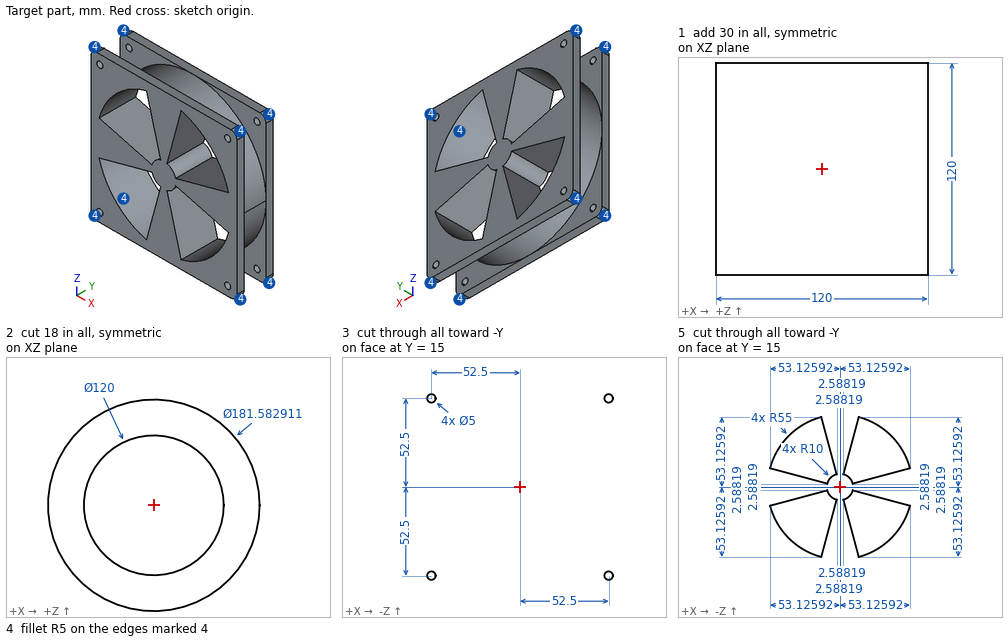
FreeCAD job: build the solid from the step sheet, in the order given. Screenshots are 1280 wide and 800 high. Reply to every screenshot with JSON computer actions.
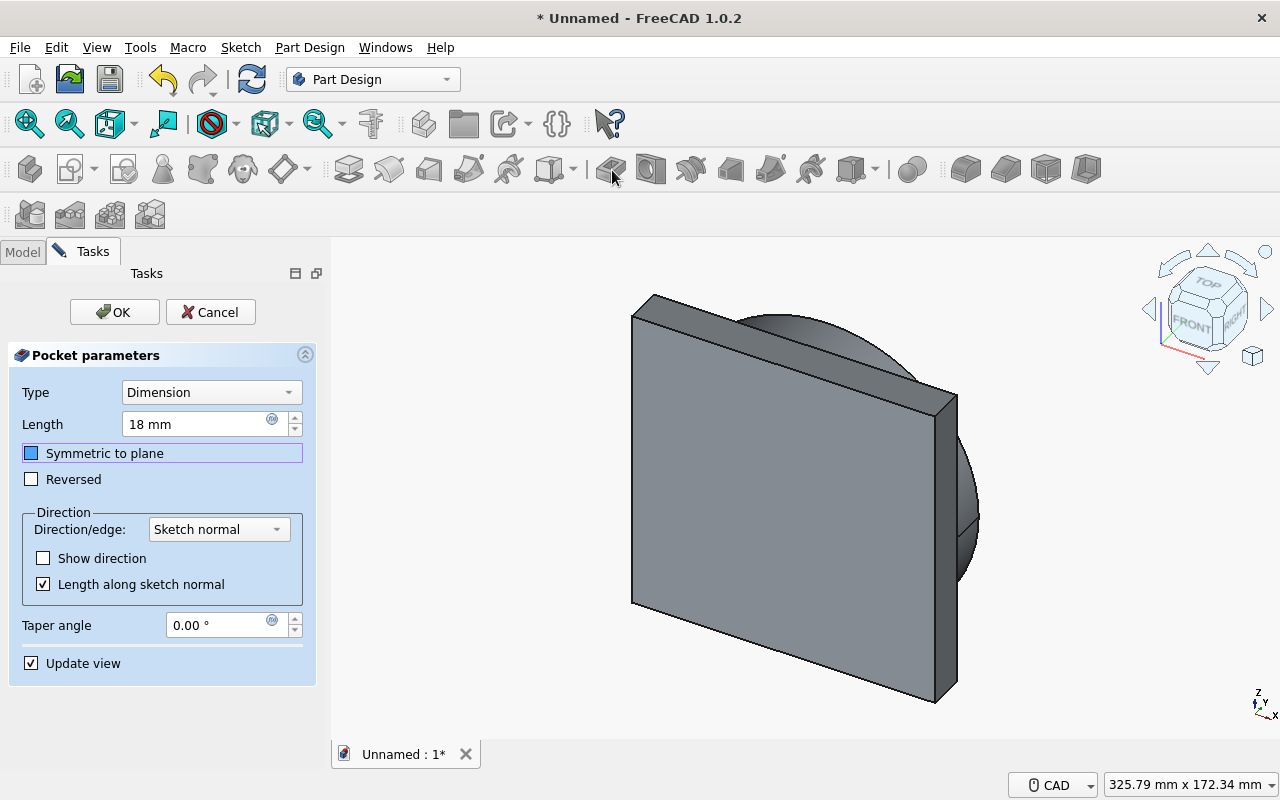
{"action": "left_click", "coordinate": [30, 453]}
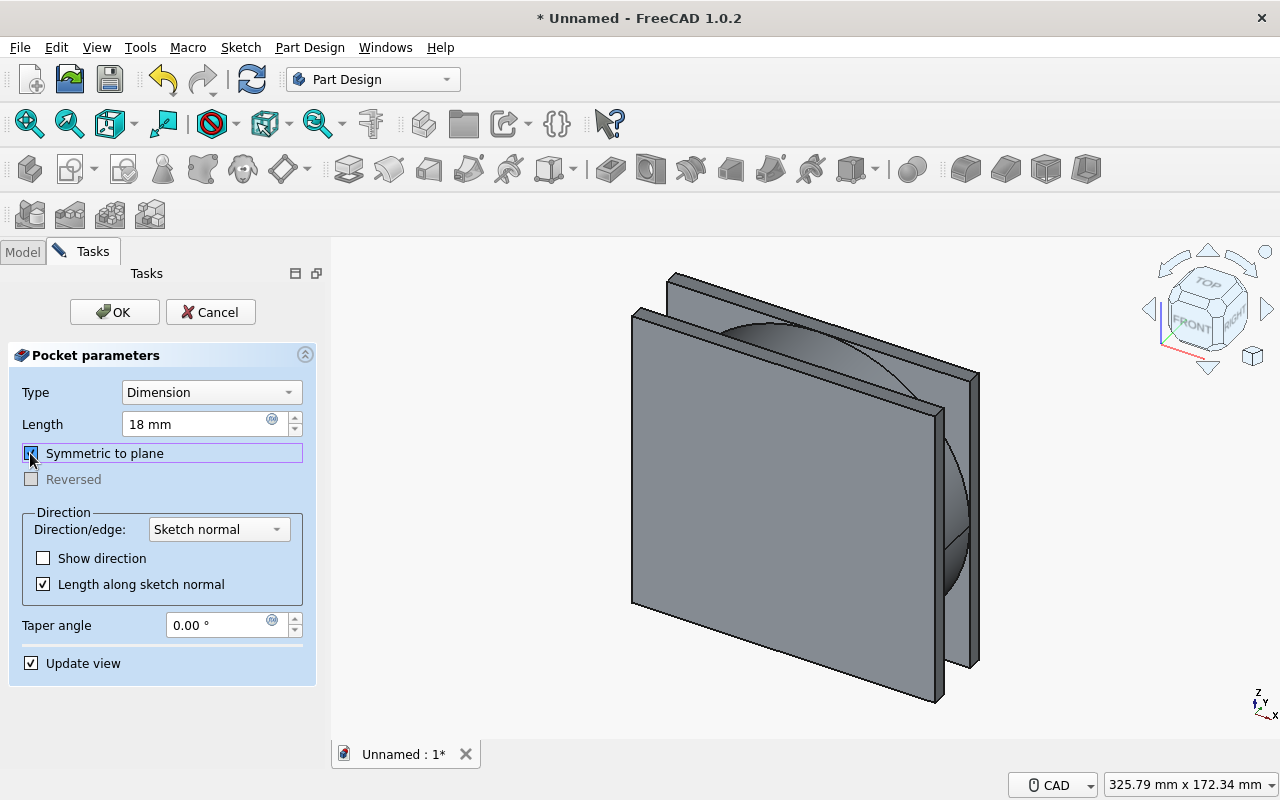
{"action": "left_click", "coordinate": [115, 312]}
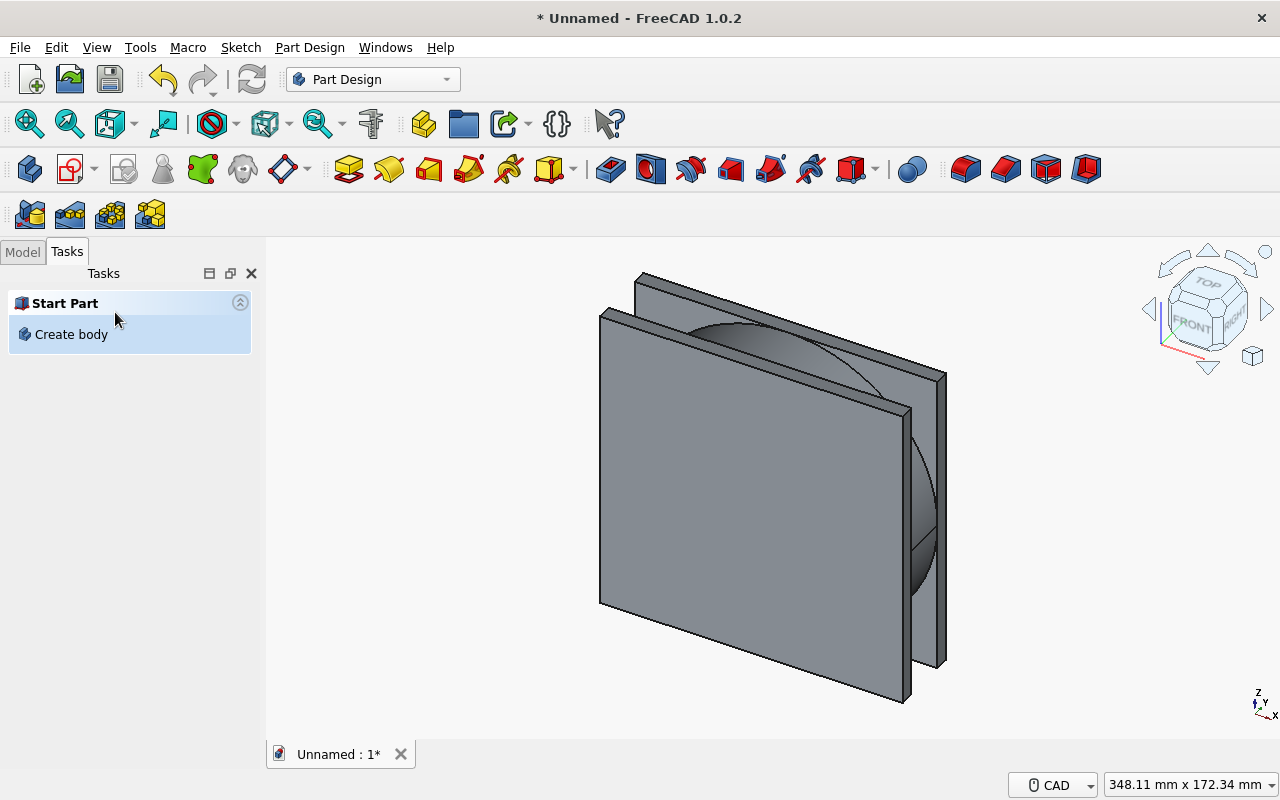
{"action": "key", "text": "4"}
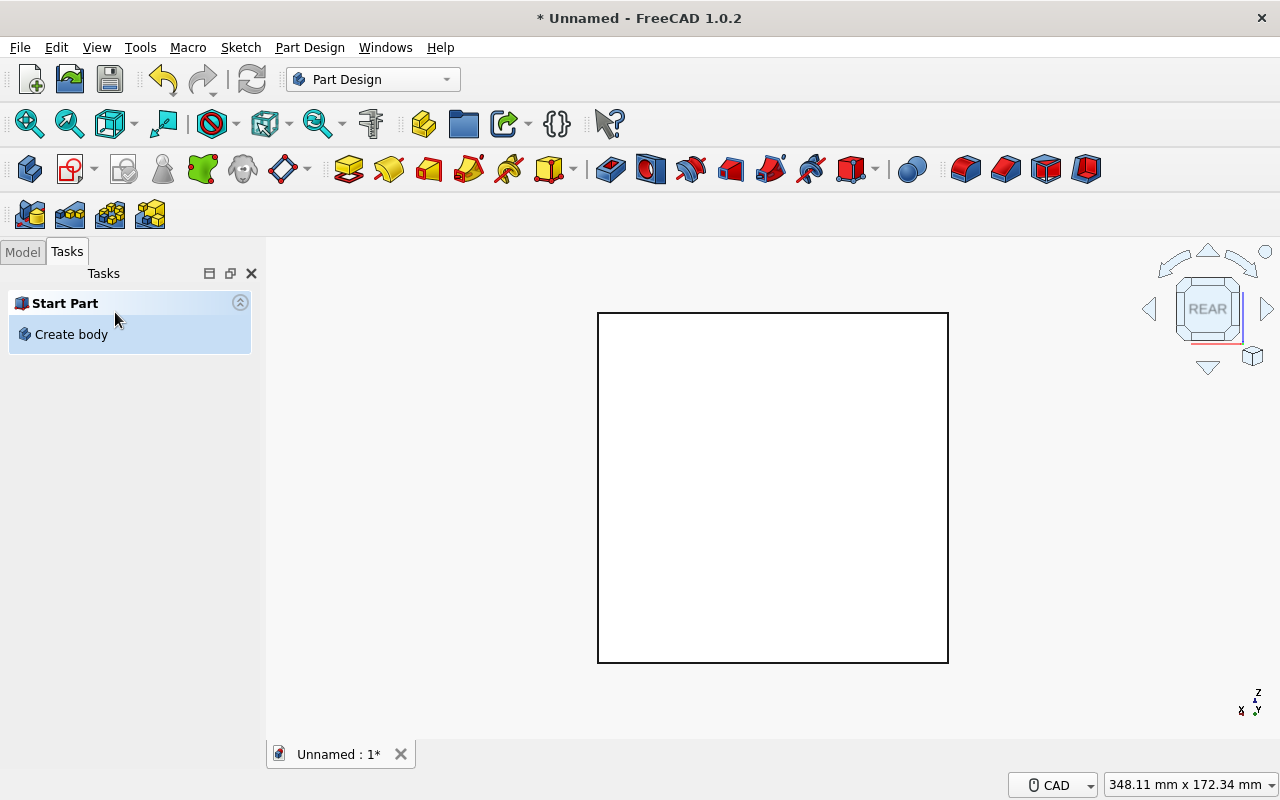
{"action": "left_click", "coordinate": [773, 487]}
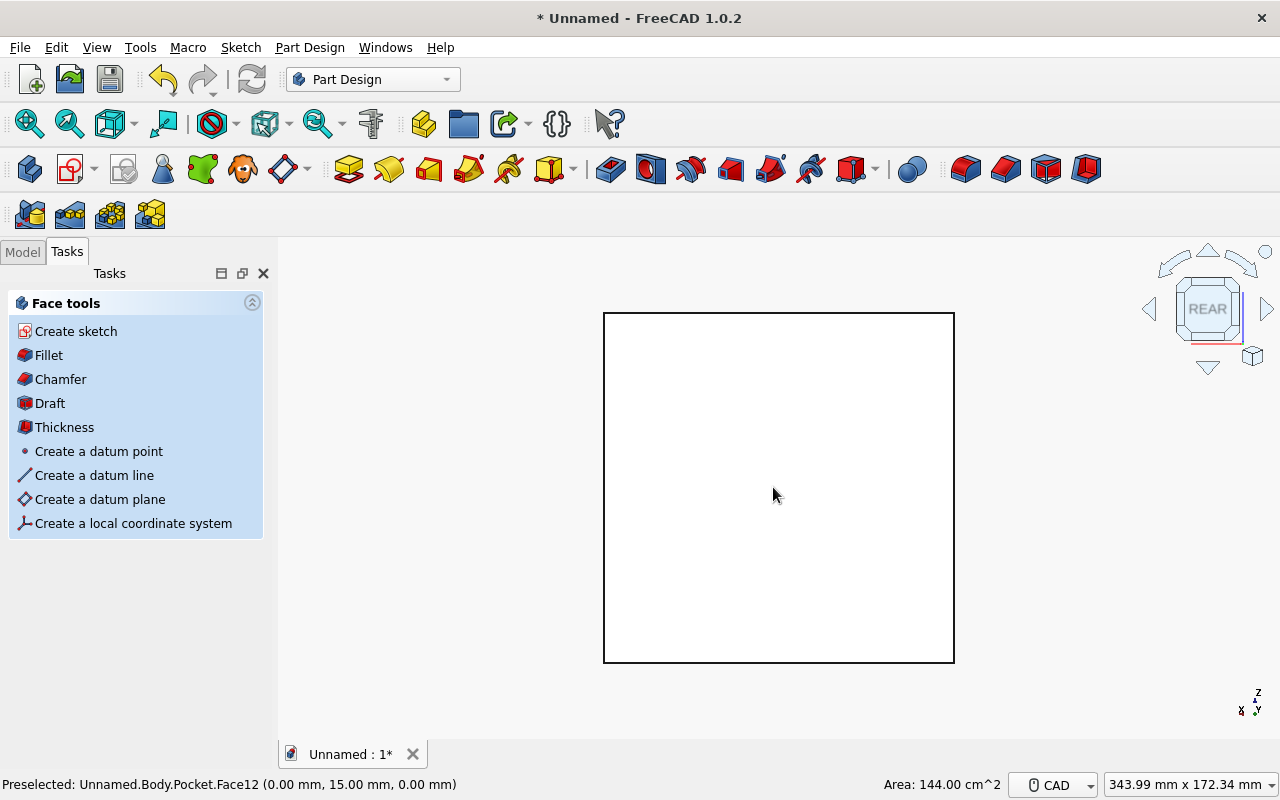
{"action": "left_click", "coordinate": [70, 170]}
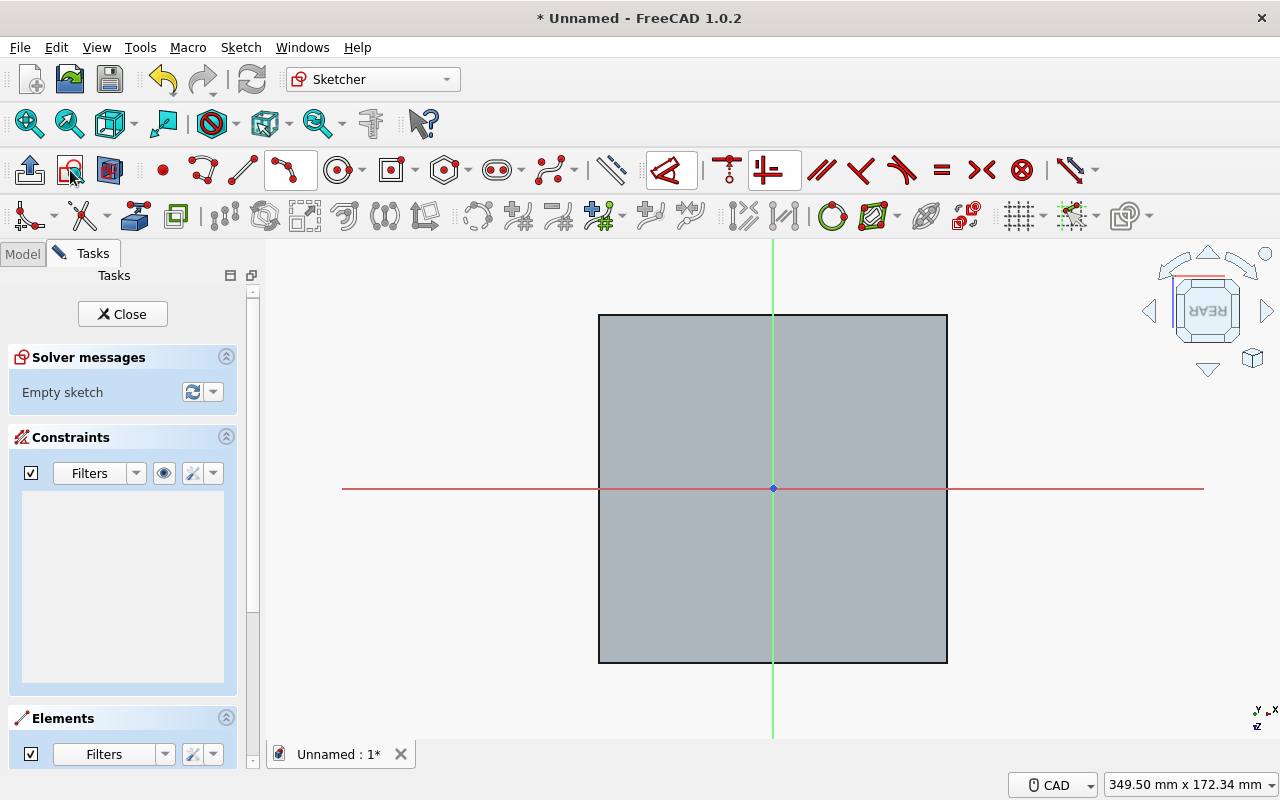
{"action": "left_click", "coordinate": [338, 170]}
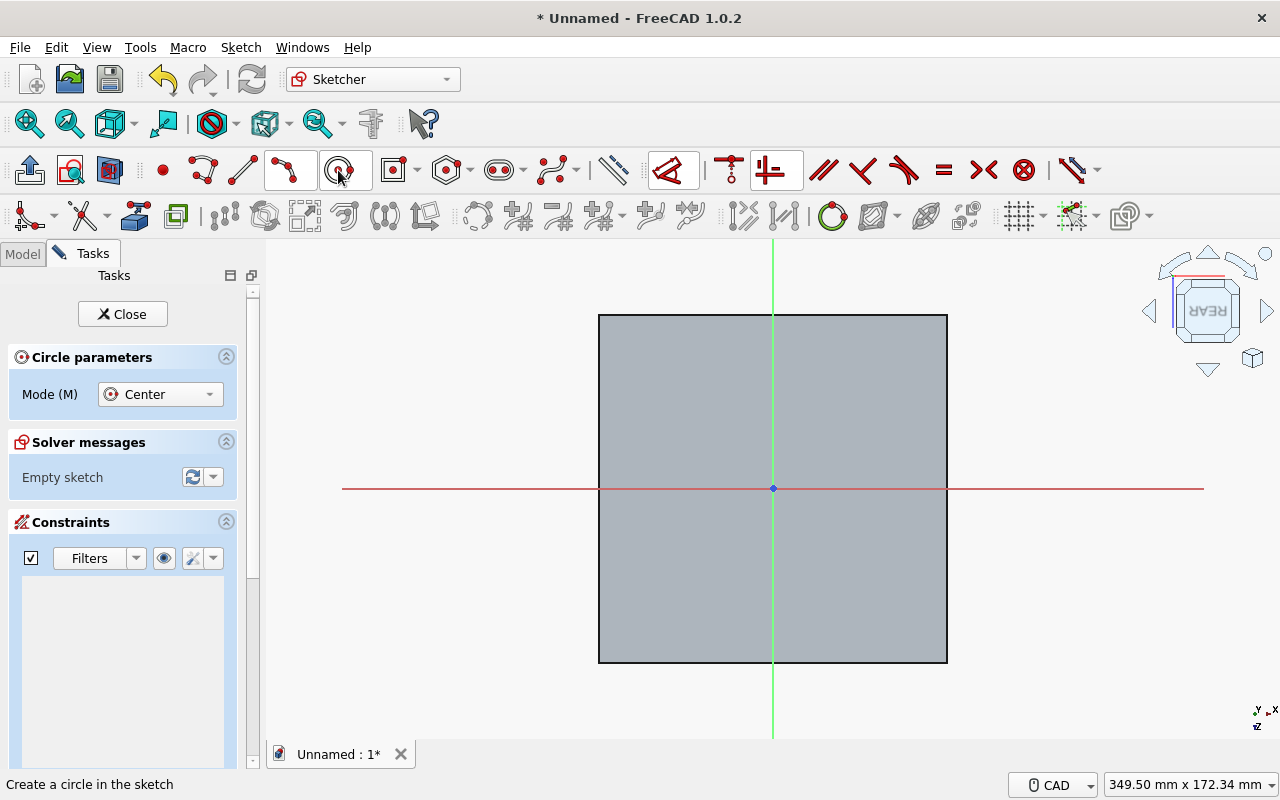
{"action": "scroll", "coordinate": [621, 337], "scroll_direction": "up", "scroll_amount": 6}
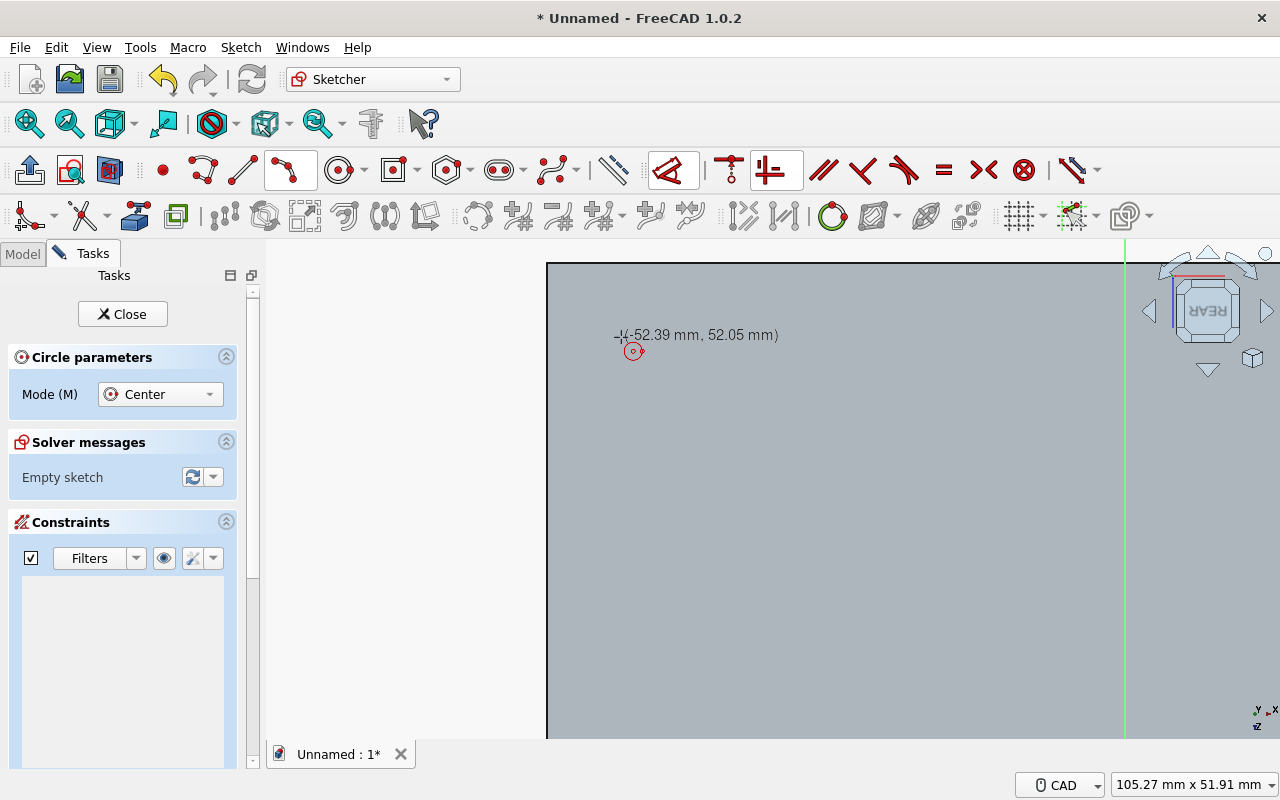
{"action": "left_click", "coordinate": [619, 335]}
{"action": "left_click", "coordinate": [636, 318]}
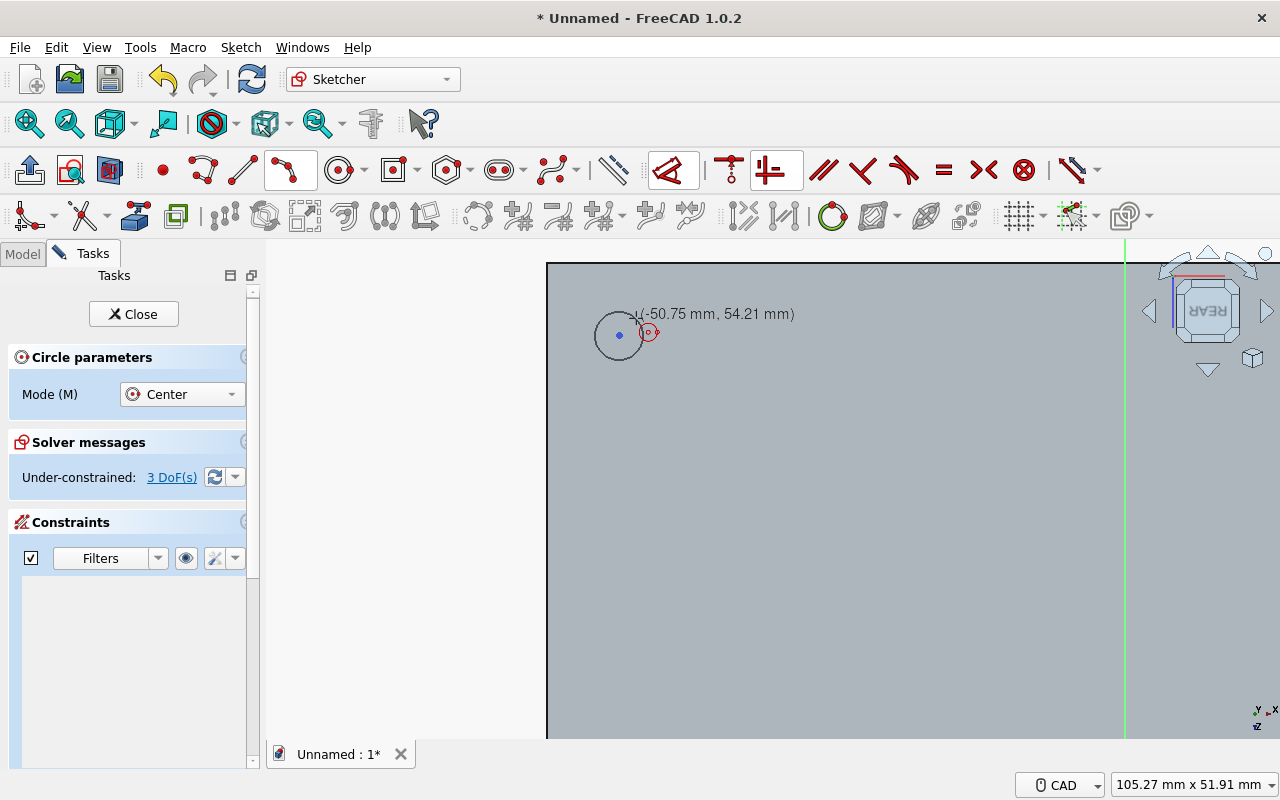
{"action": "scroll", "coordinate": [523, 337], "scroll_direction": "down", "scroll_amount": 6}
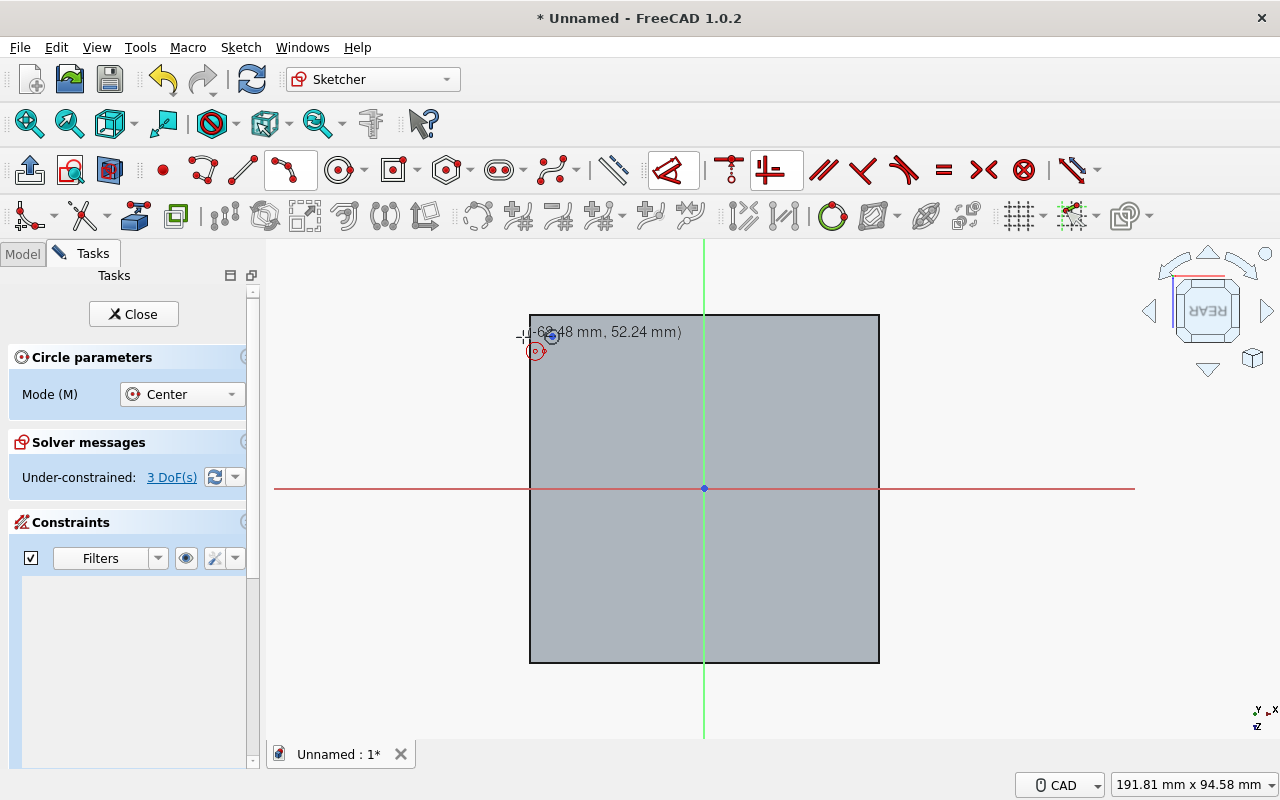
{"action": "scroll", "coordinate": [552, 641], "scroll_direction": "up", "scroll_amount": 6}